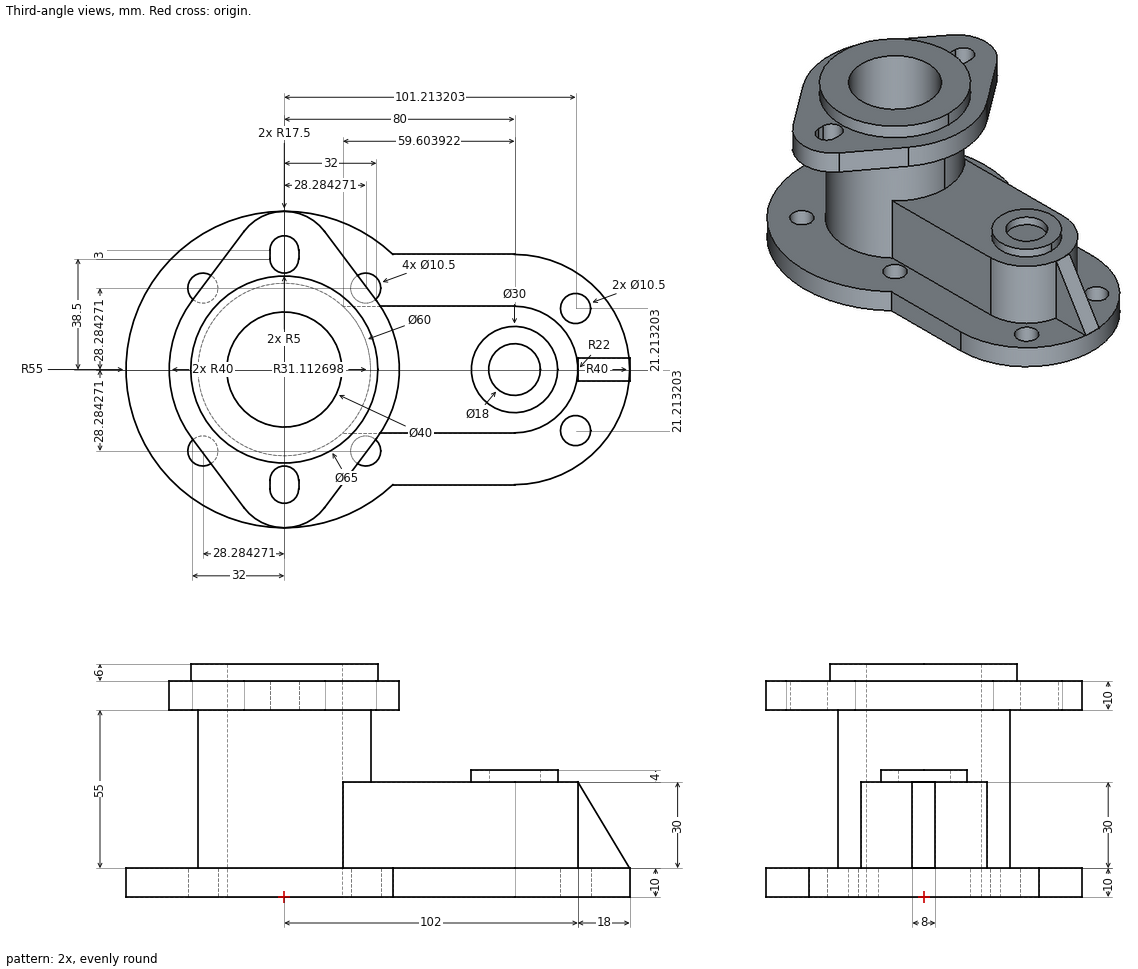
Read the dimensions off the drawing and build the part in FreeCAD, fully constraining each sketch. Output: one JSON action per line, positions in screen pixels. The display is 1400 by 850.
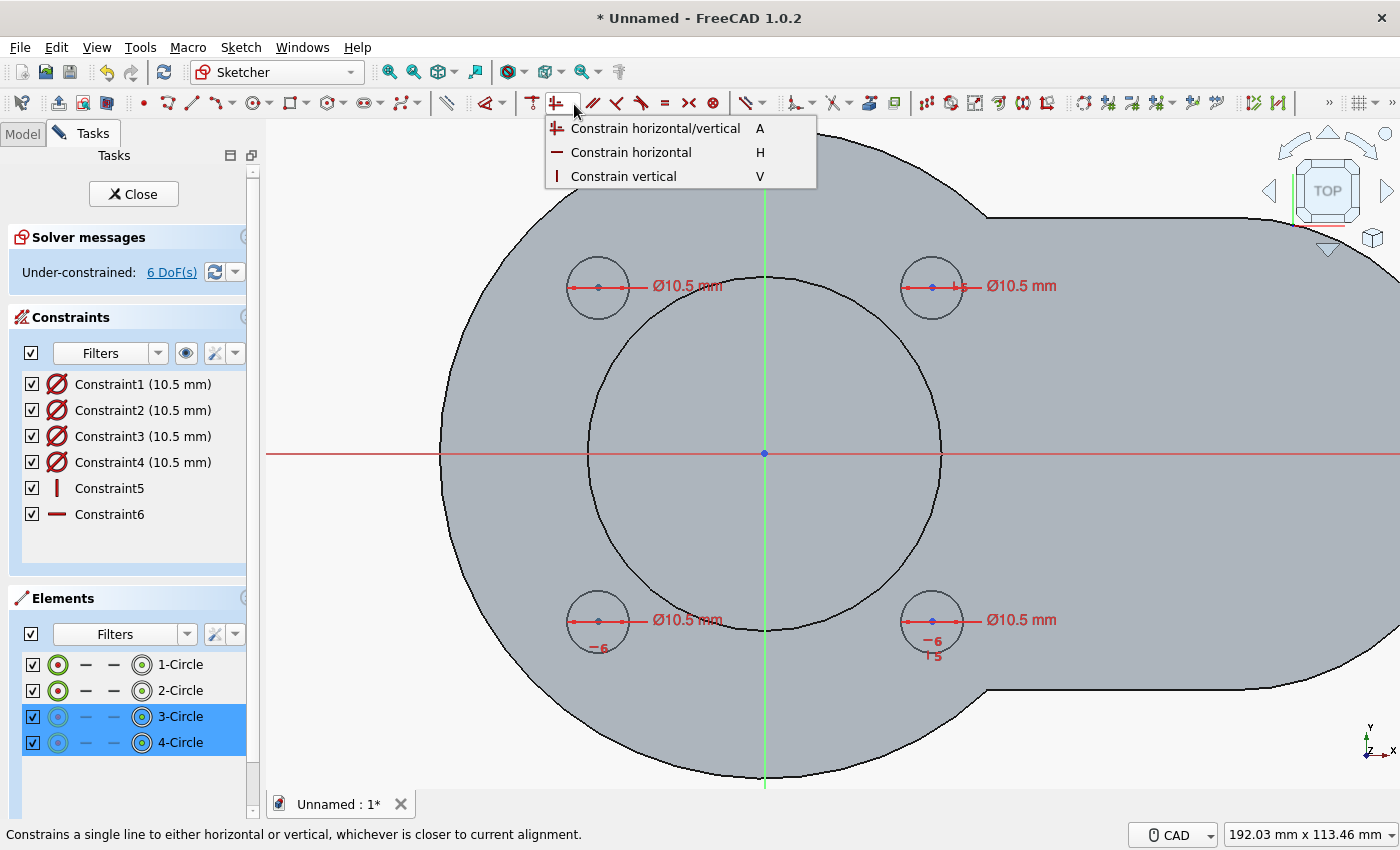
{"action": "left_click", "coordinate": [681, 176]}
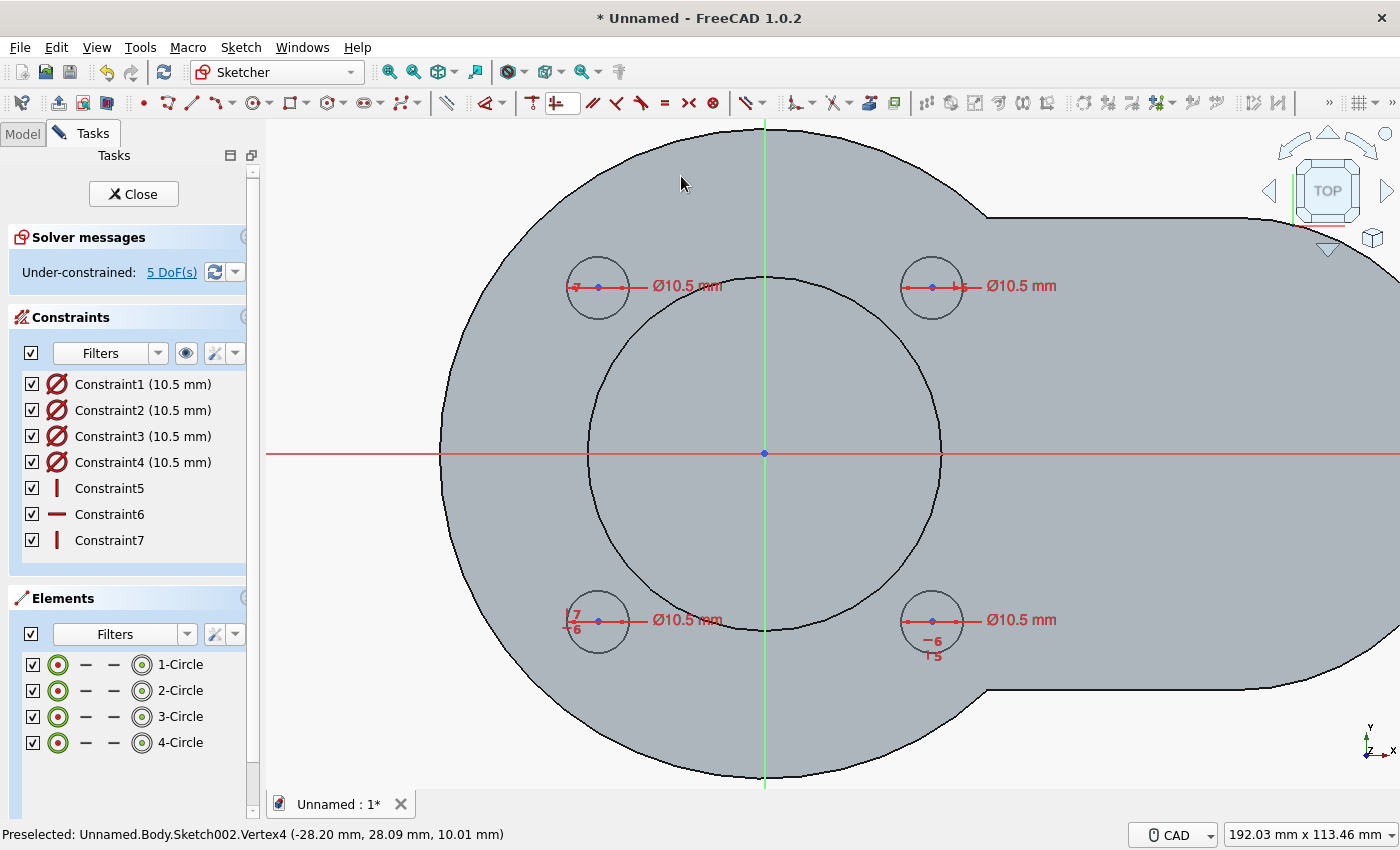
{"action": "left_click", "coordinate": [932, 288]}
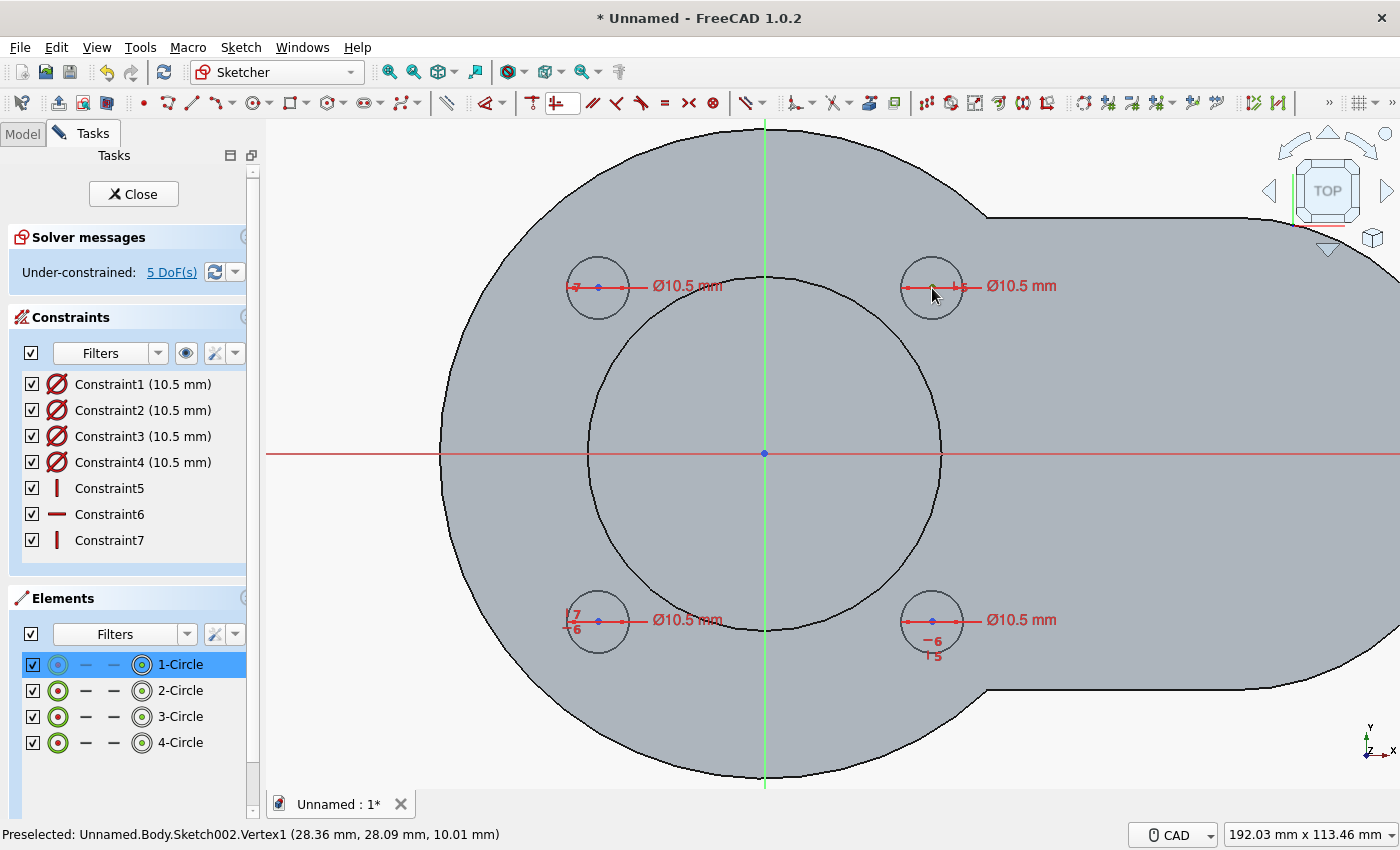
{"action": "left_click", "coordinate": [598, 288]}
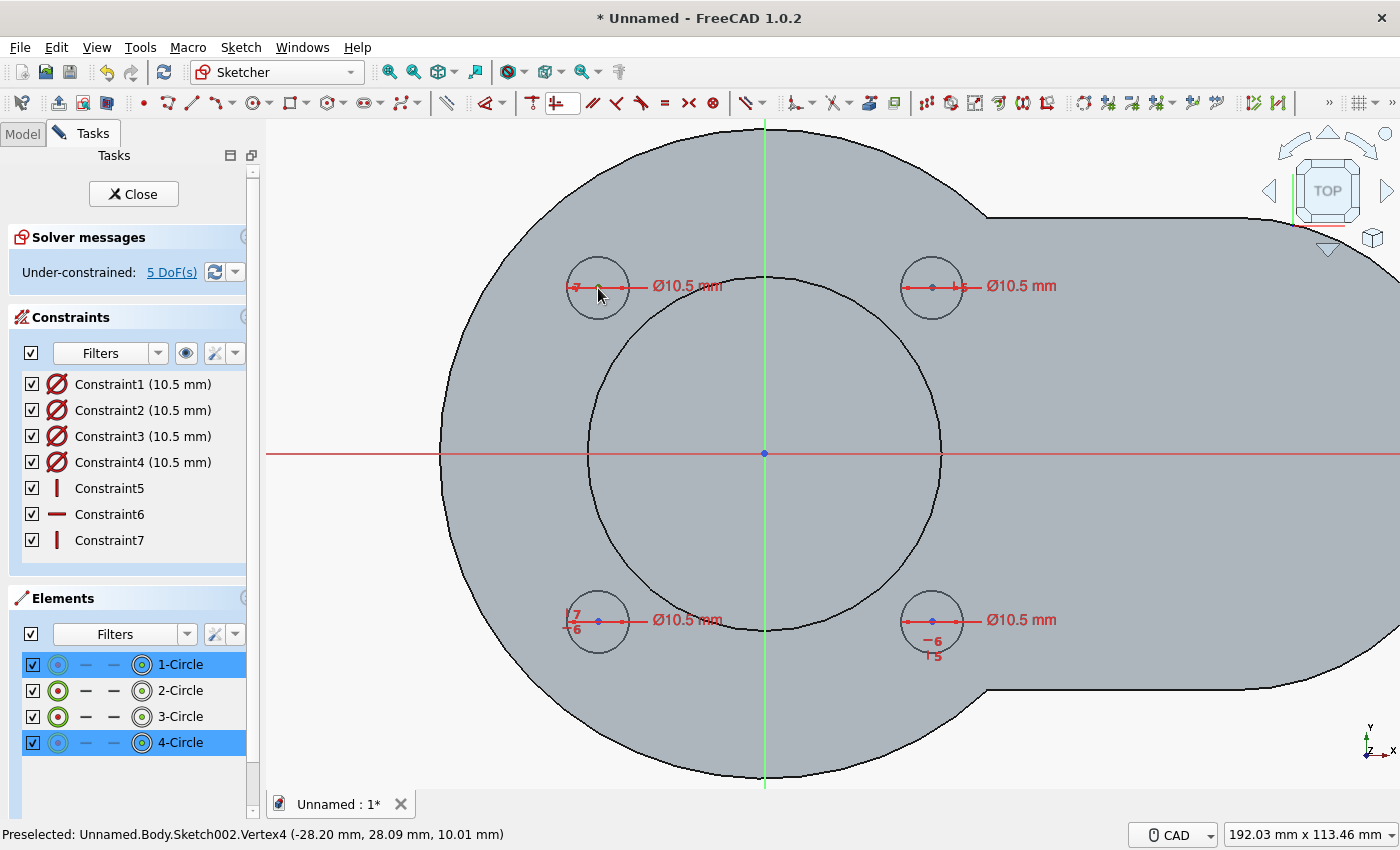
{"action": "left_click", "coordinate": [574, 104]}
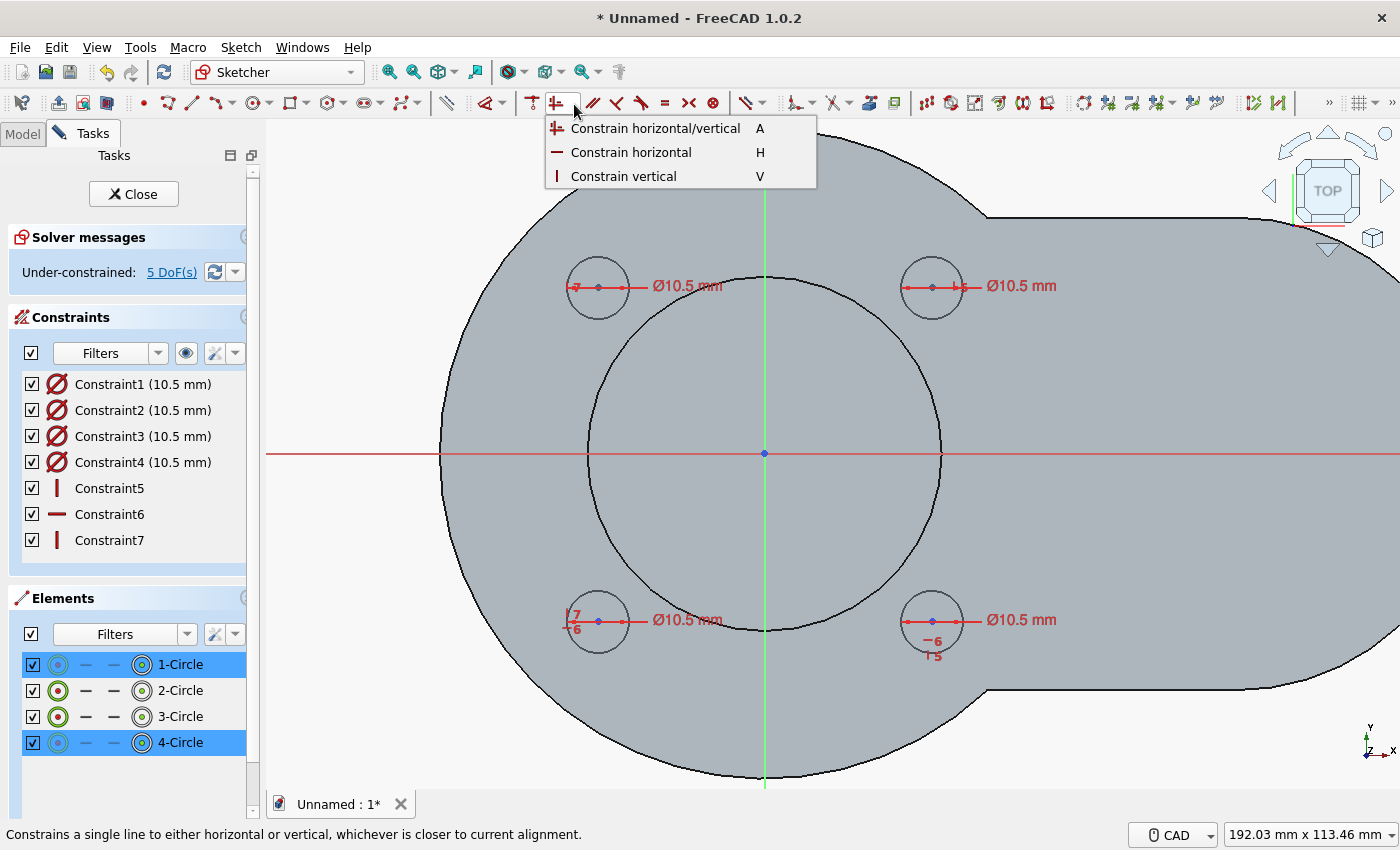
{"action": "left_click", "coordinate": [681, 152]}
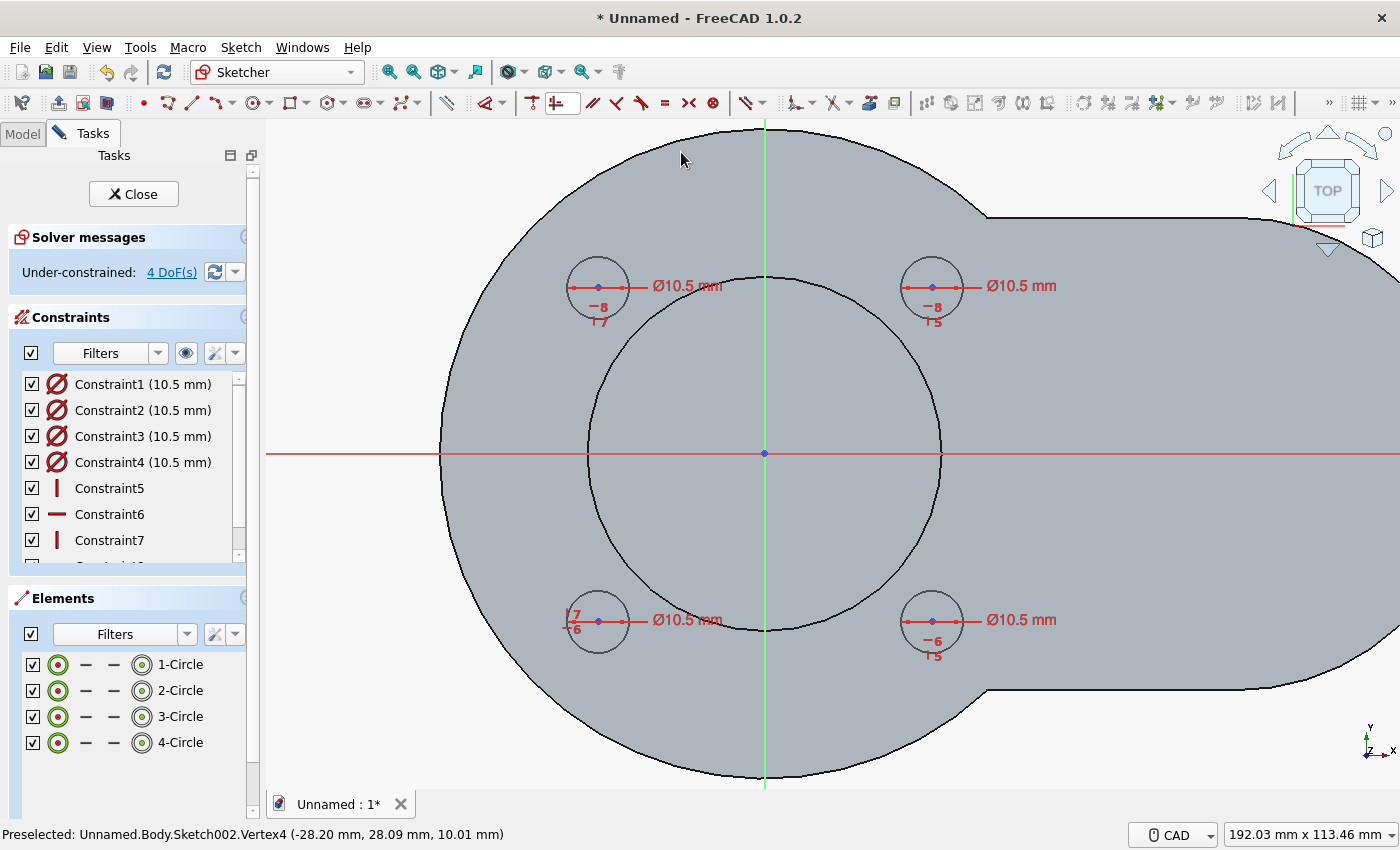
{"action": "left_click", "coordinate": [486, 104]}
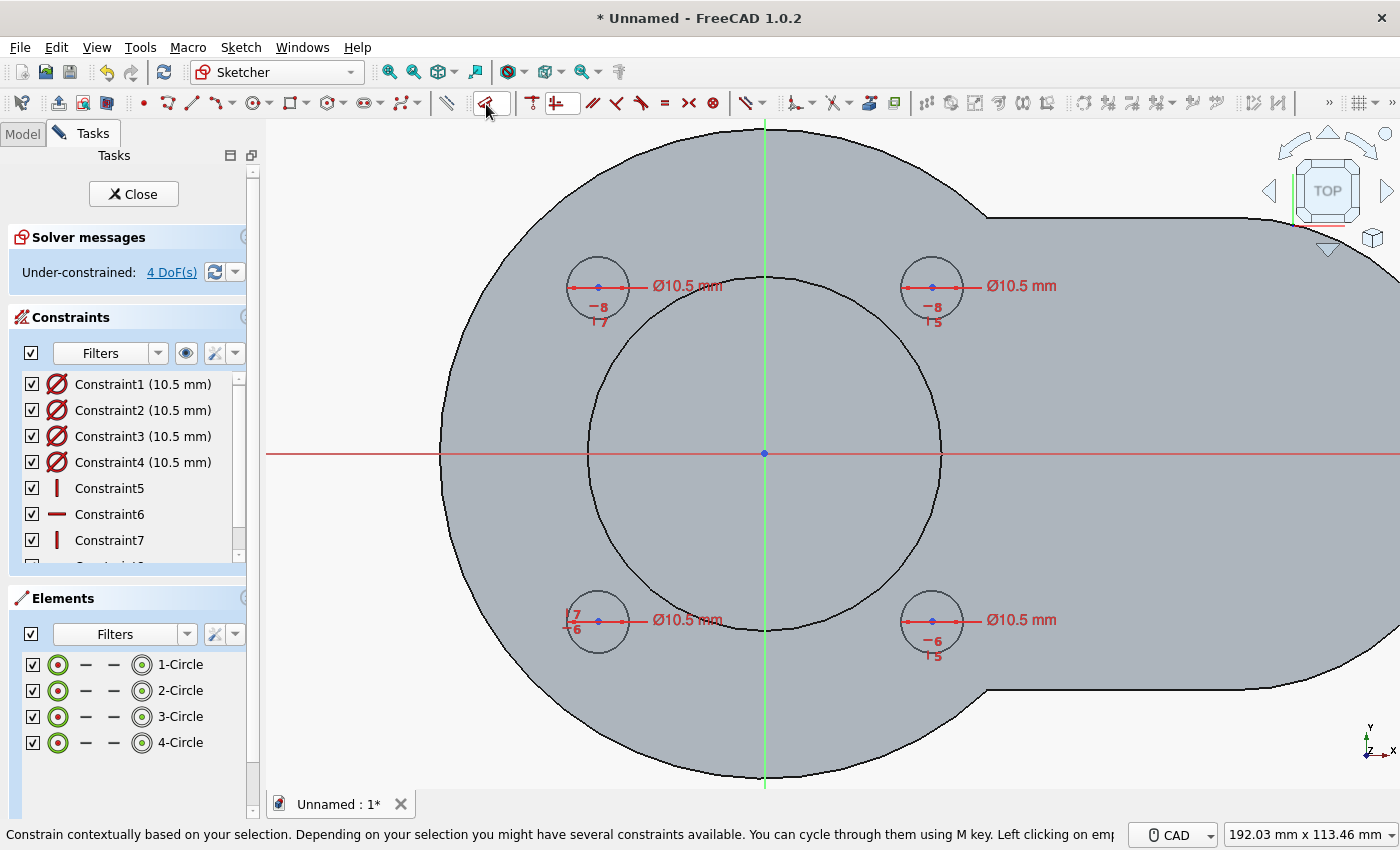
{"action": "left_click", "coordinate": [932, 288]}
{"action": "left_click", "coordinate": [848, 254]}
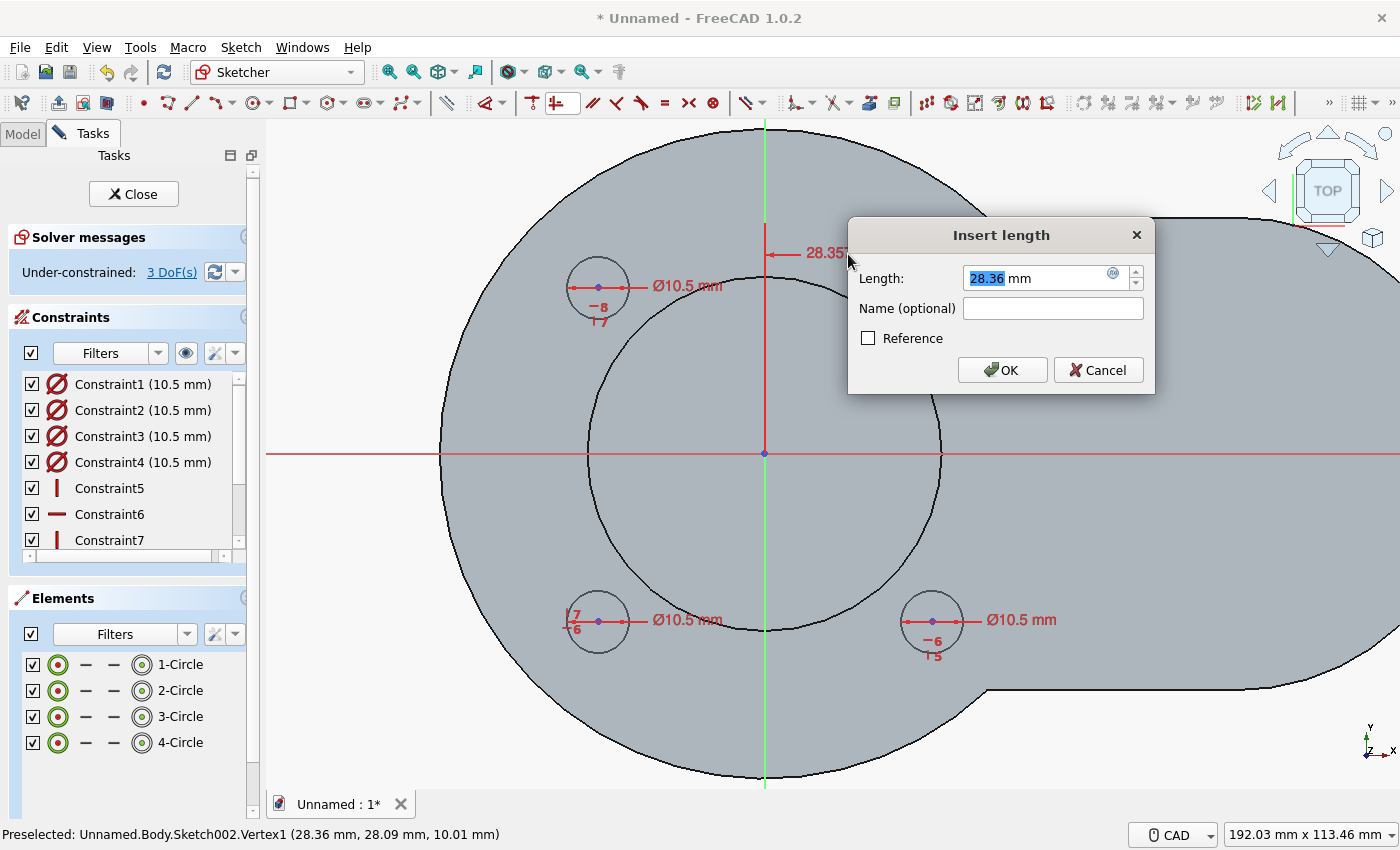
{"action": "type", "text": "28.284271"}
{"action": "key", "text": "Return"}